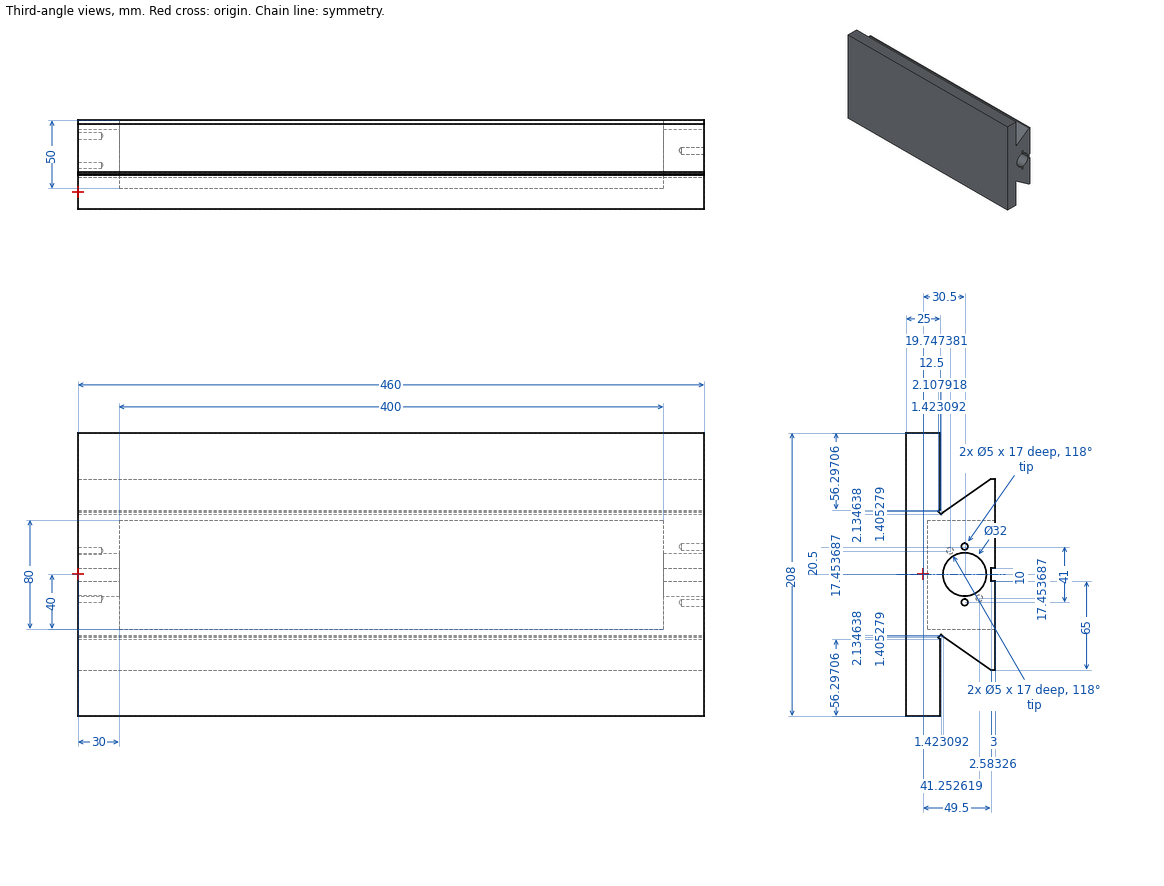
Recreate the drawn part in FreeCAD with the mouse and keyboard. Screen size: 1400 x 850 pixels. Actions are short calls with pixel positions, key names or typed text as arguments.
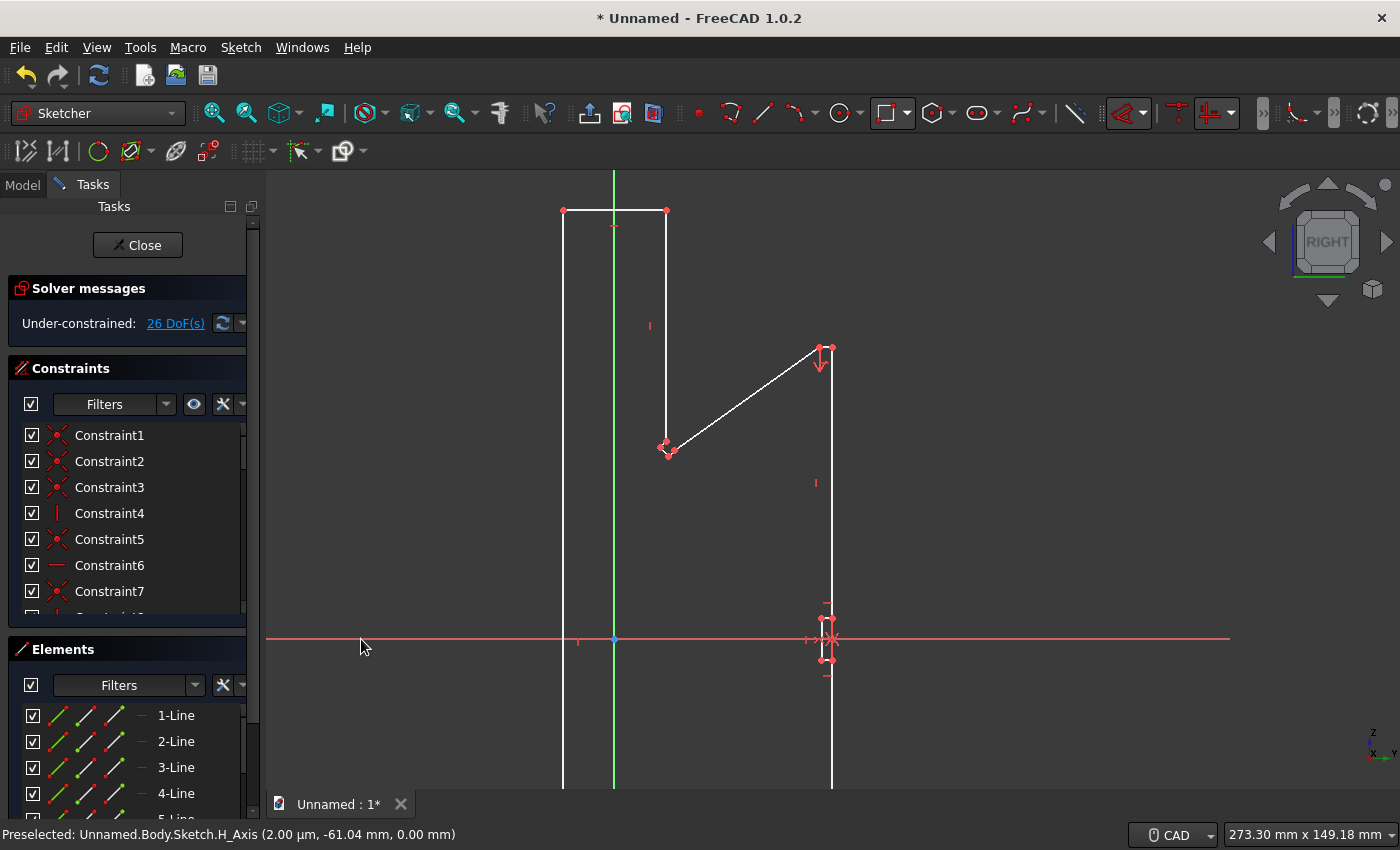
scroll(819, 349, down, 4)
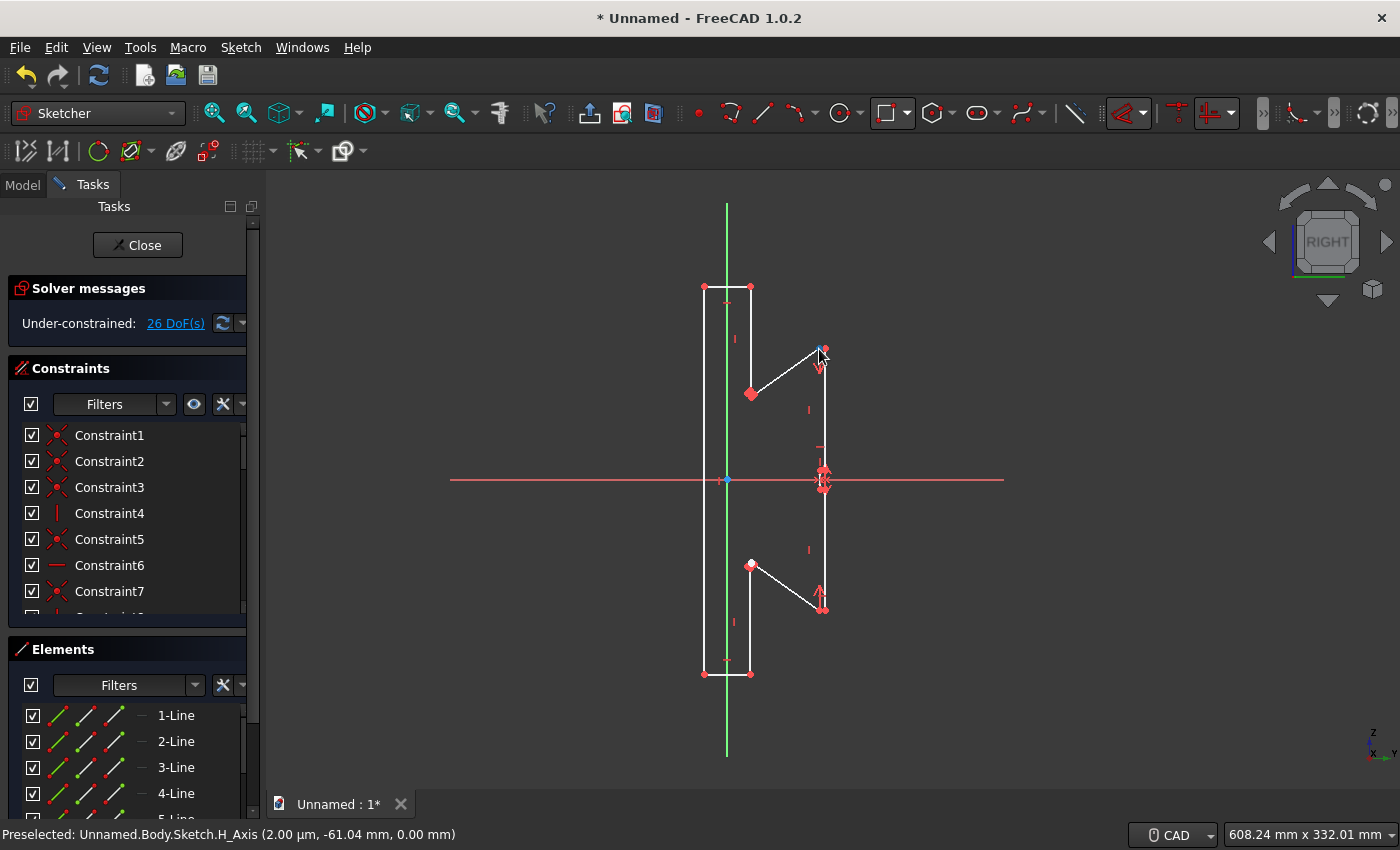
scroll(754, 565, up, 7)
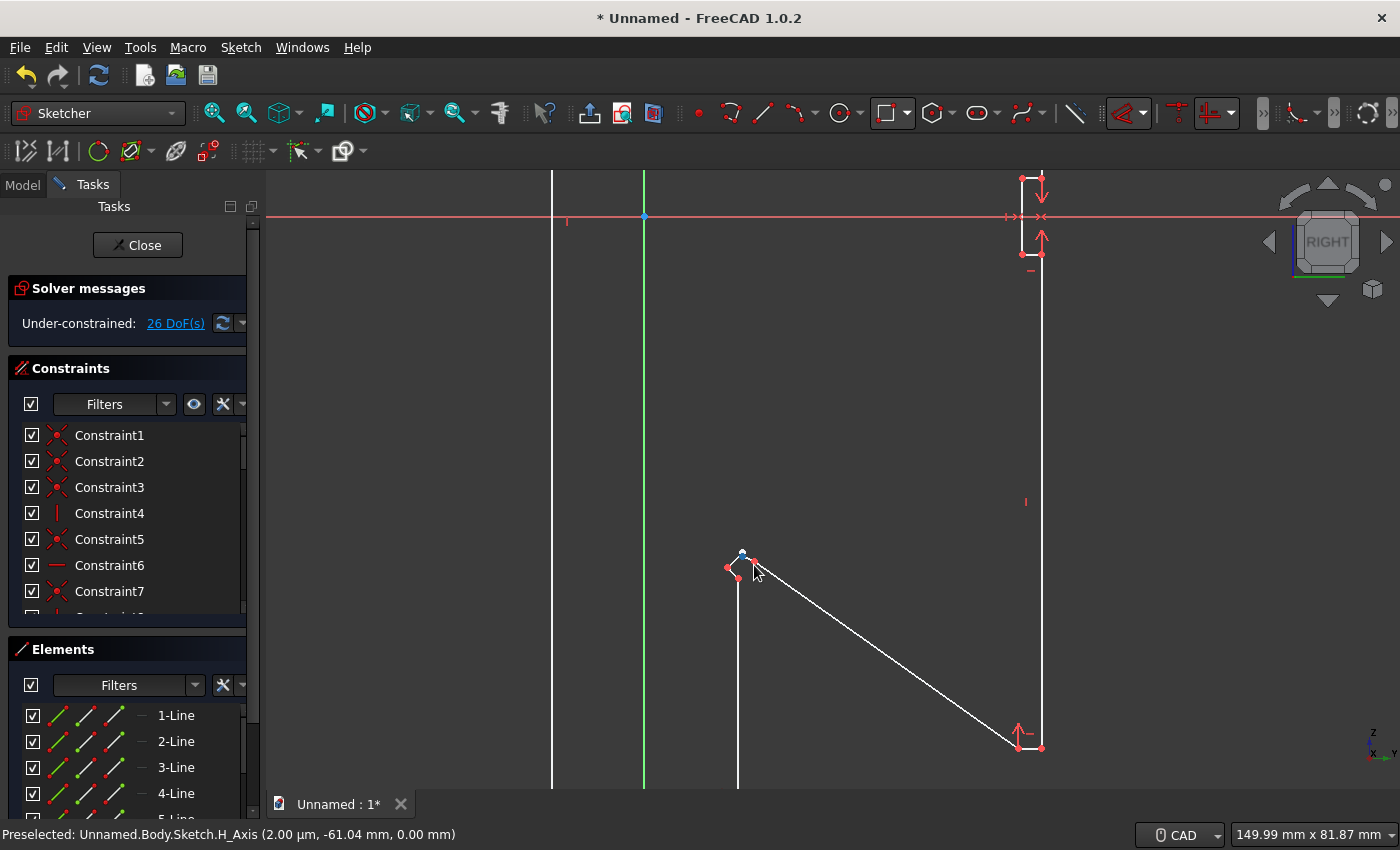
click(755, 562)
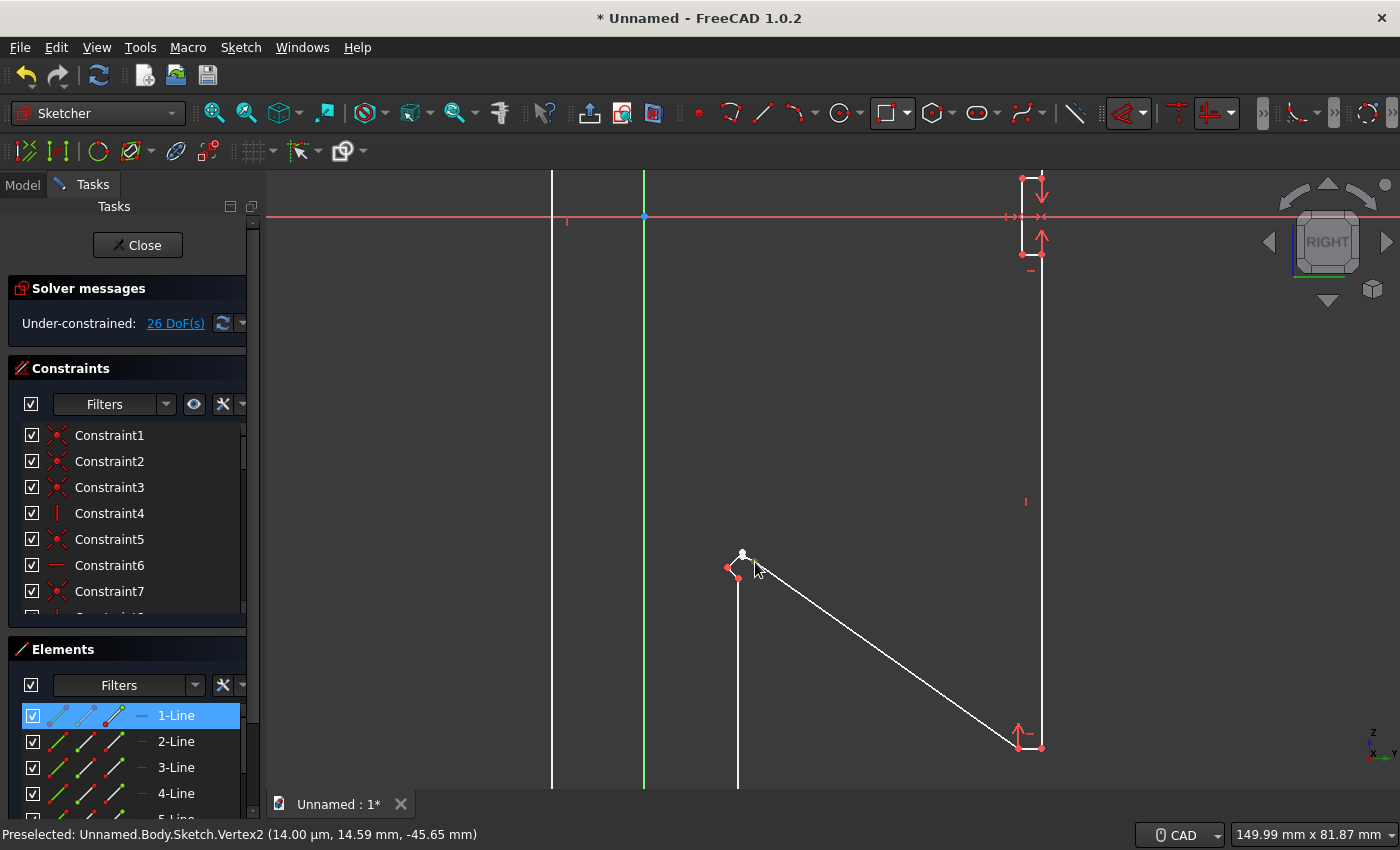
scroll(754, 566, down, 7)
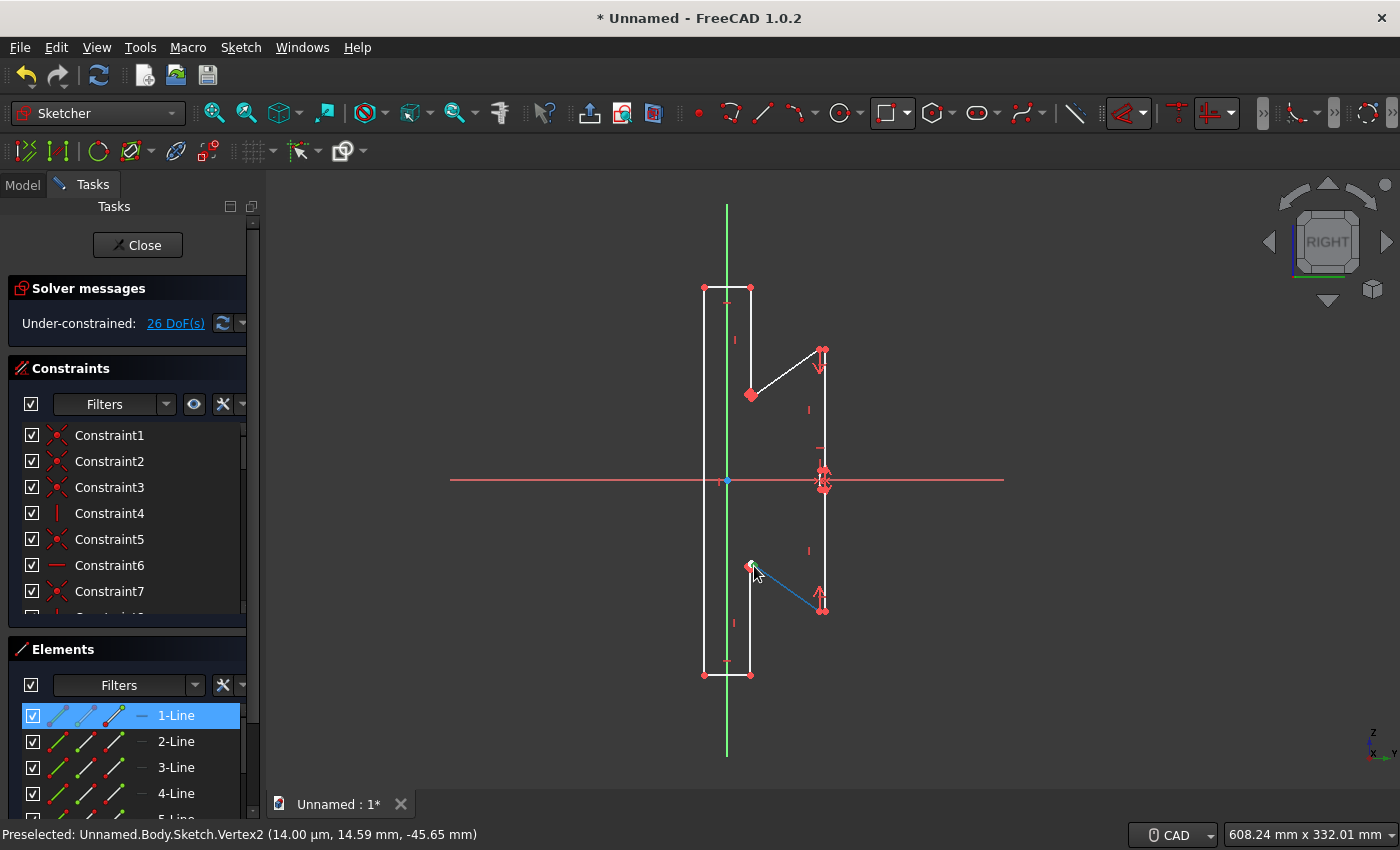
scroll(754, 396, up, 6)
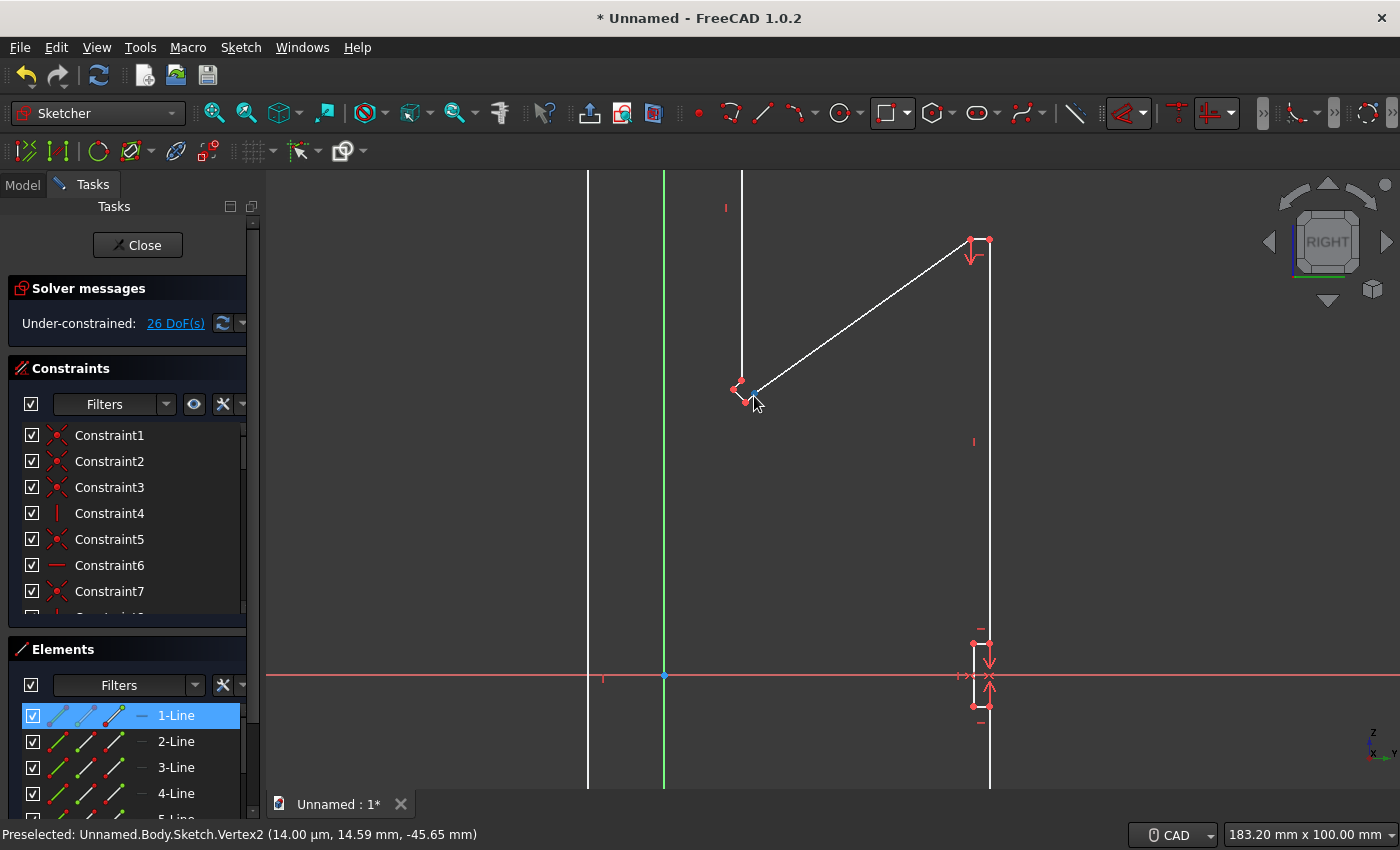
click(754, 394)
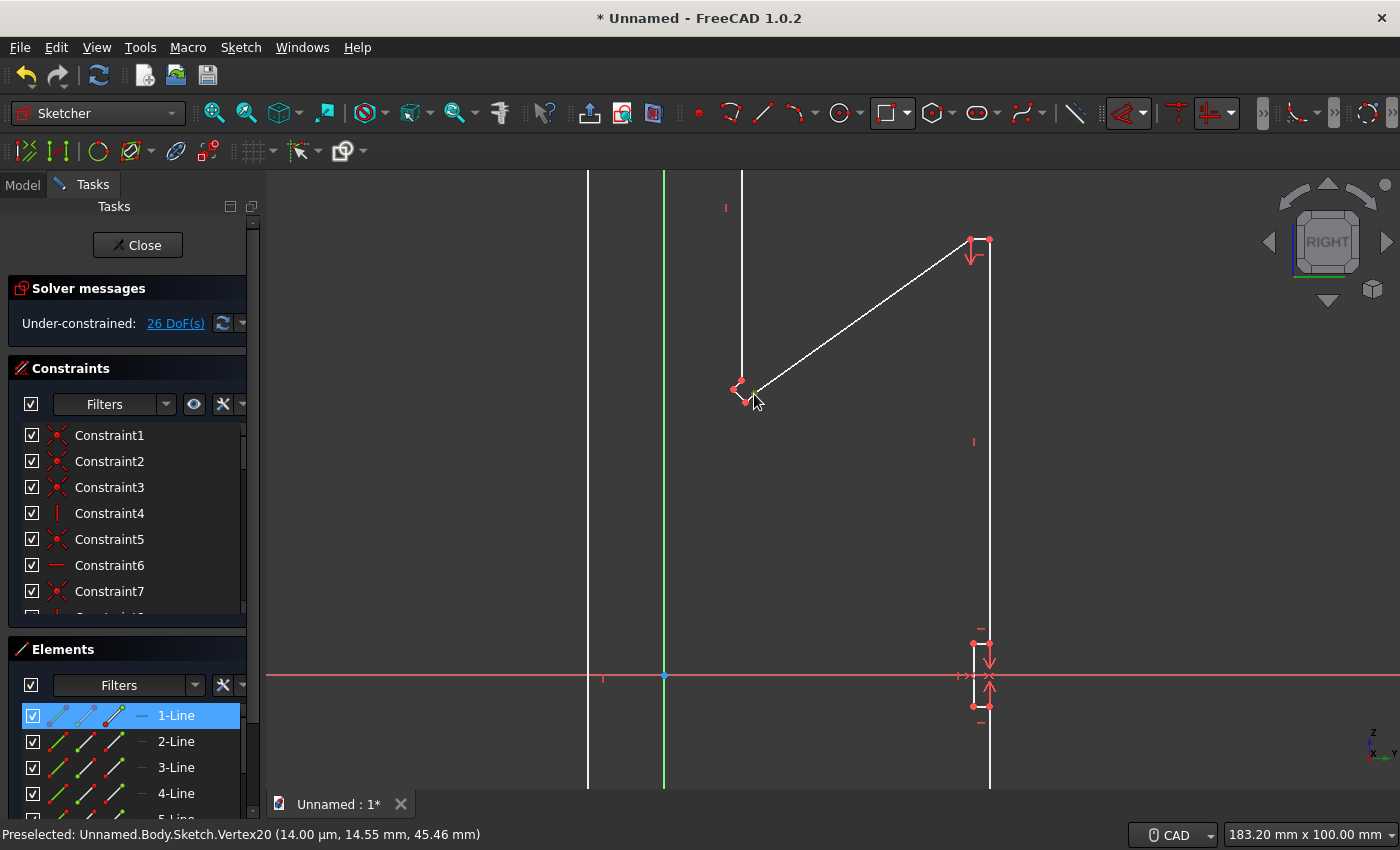
click(361, 675)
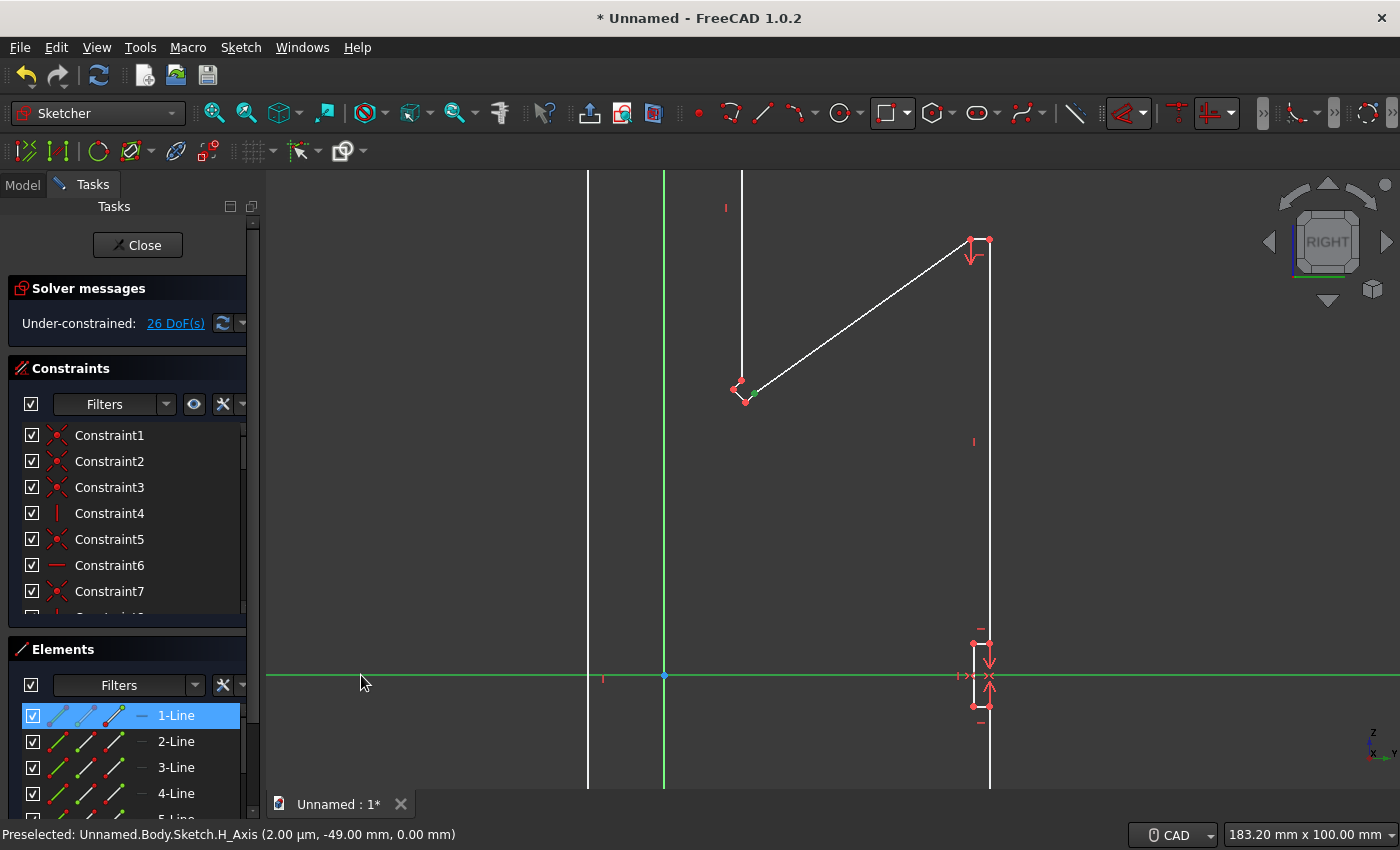
key(s)